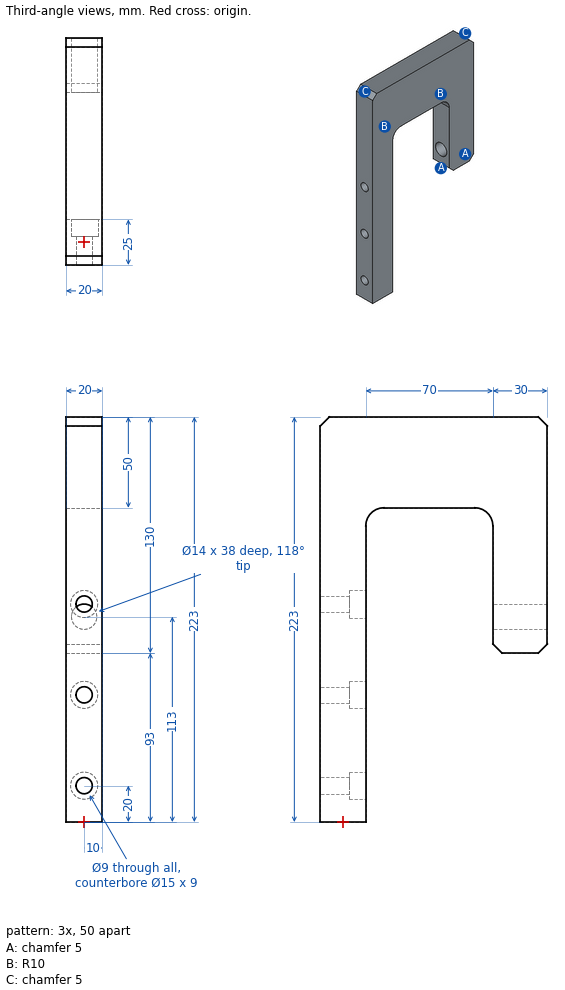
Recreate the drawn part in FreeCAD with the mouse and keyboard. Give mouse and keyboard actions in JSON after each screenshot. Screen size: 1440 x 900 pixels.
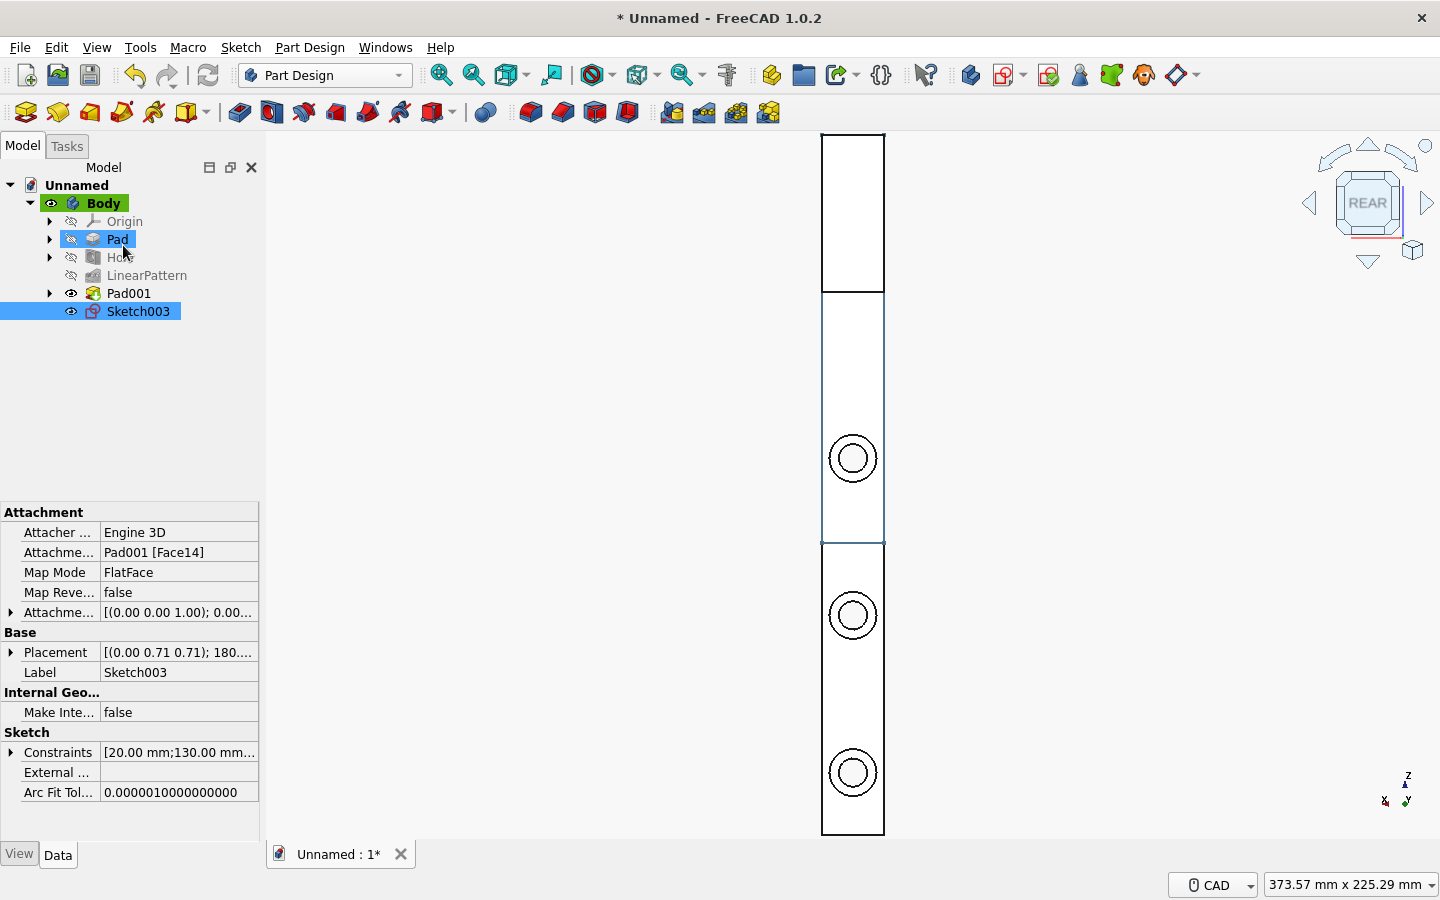
{"action": "left_click", "coordinate": [26, 112]}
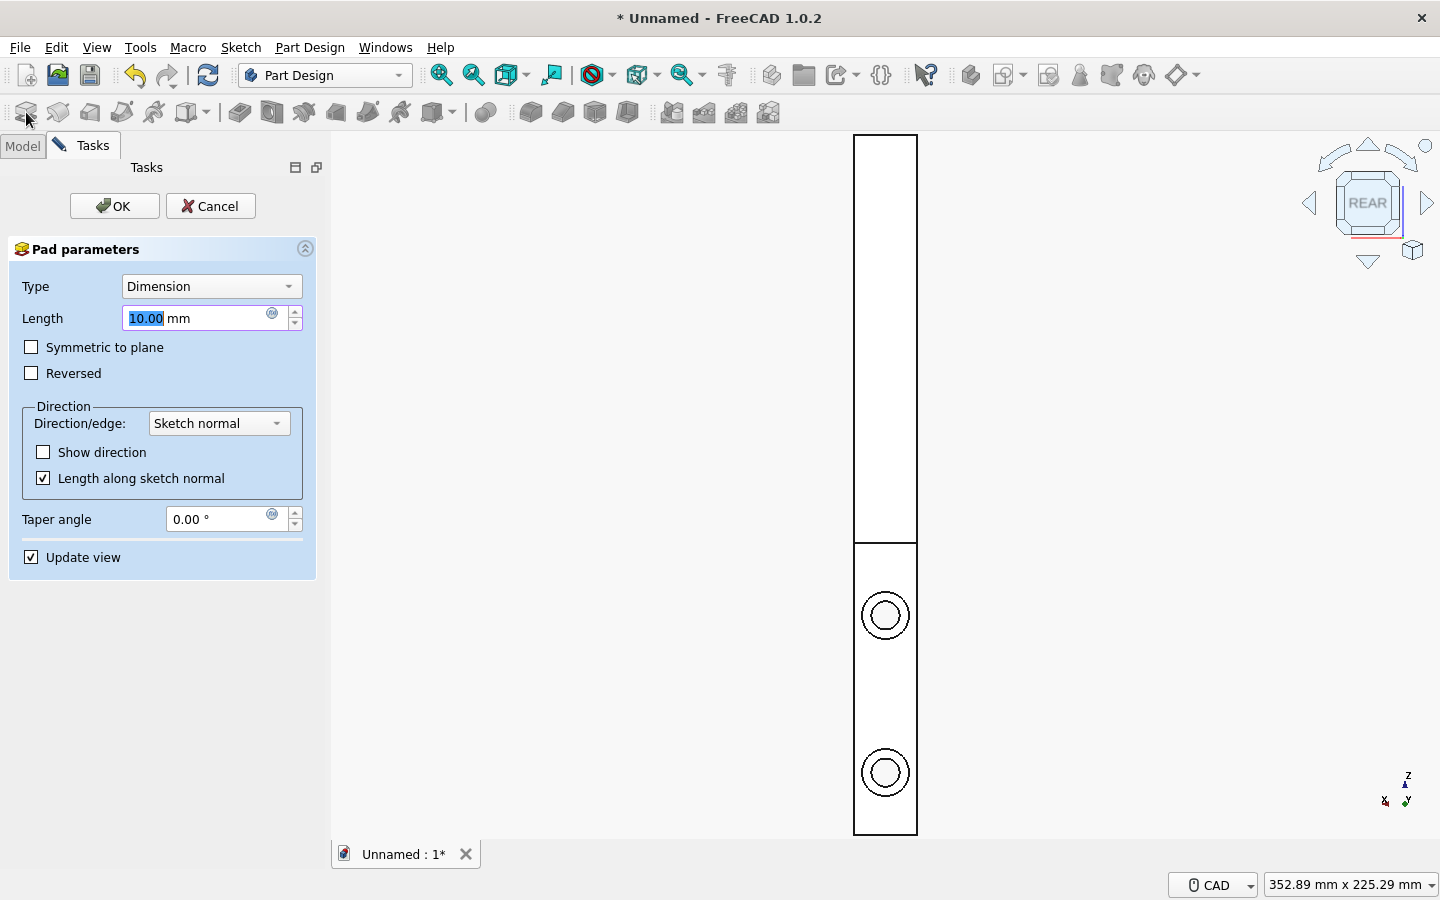
{"action": "type", "text": "30"}
{"action": "key", "text": "Tab"}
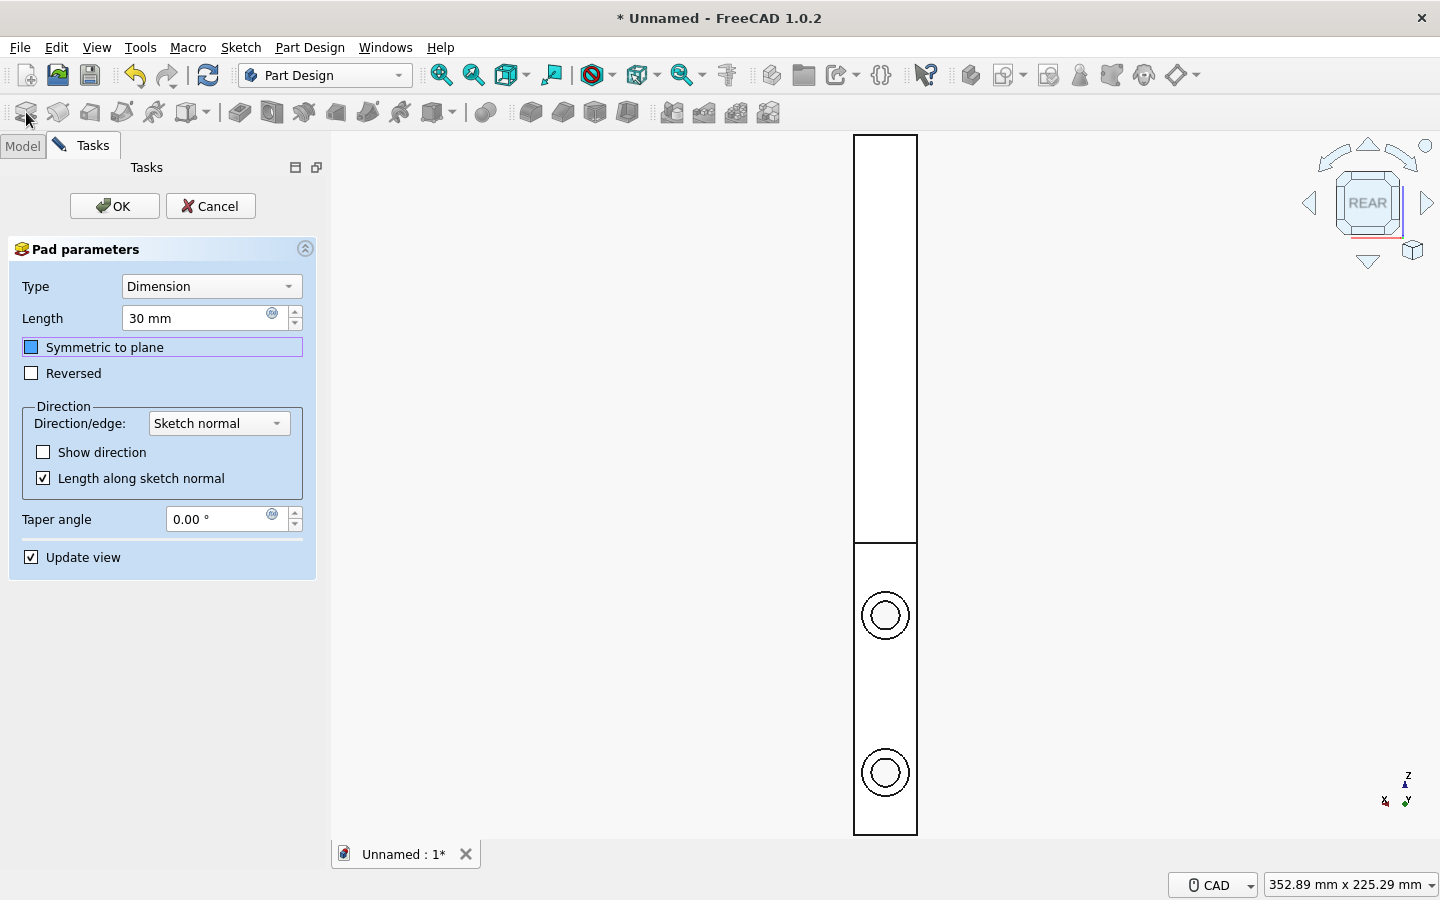
{"action": "left_click", "coordinate": [115, 206]}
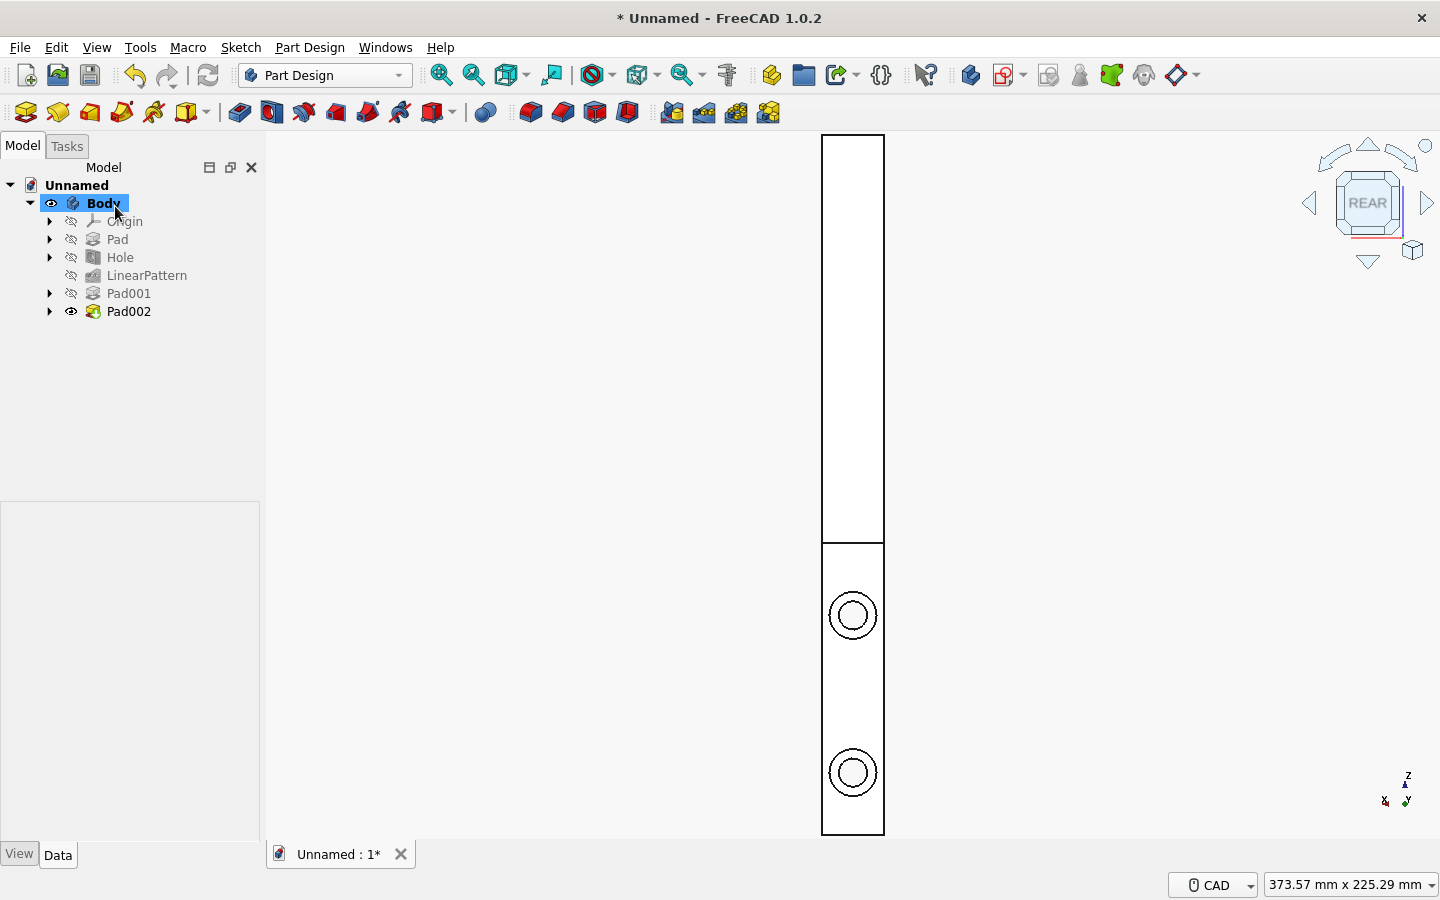
{"action": "left_click", "coordinate": [853, 221]}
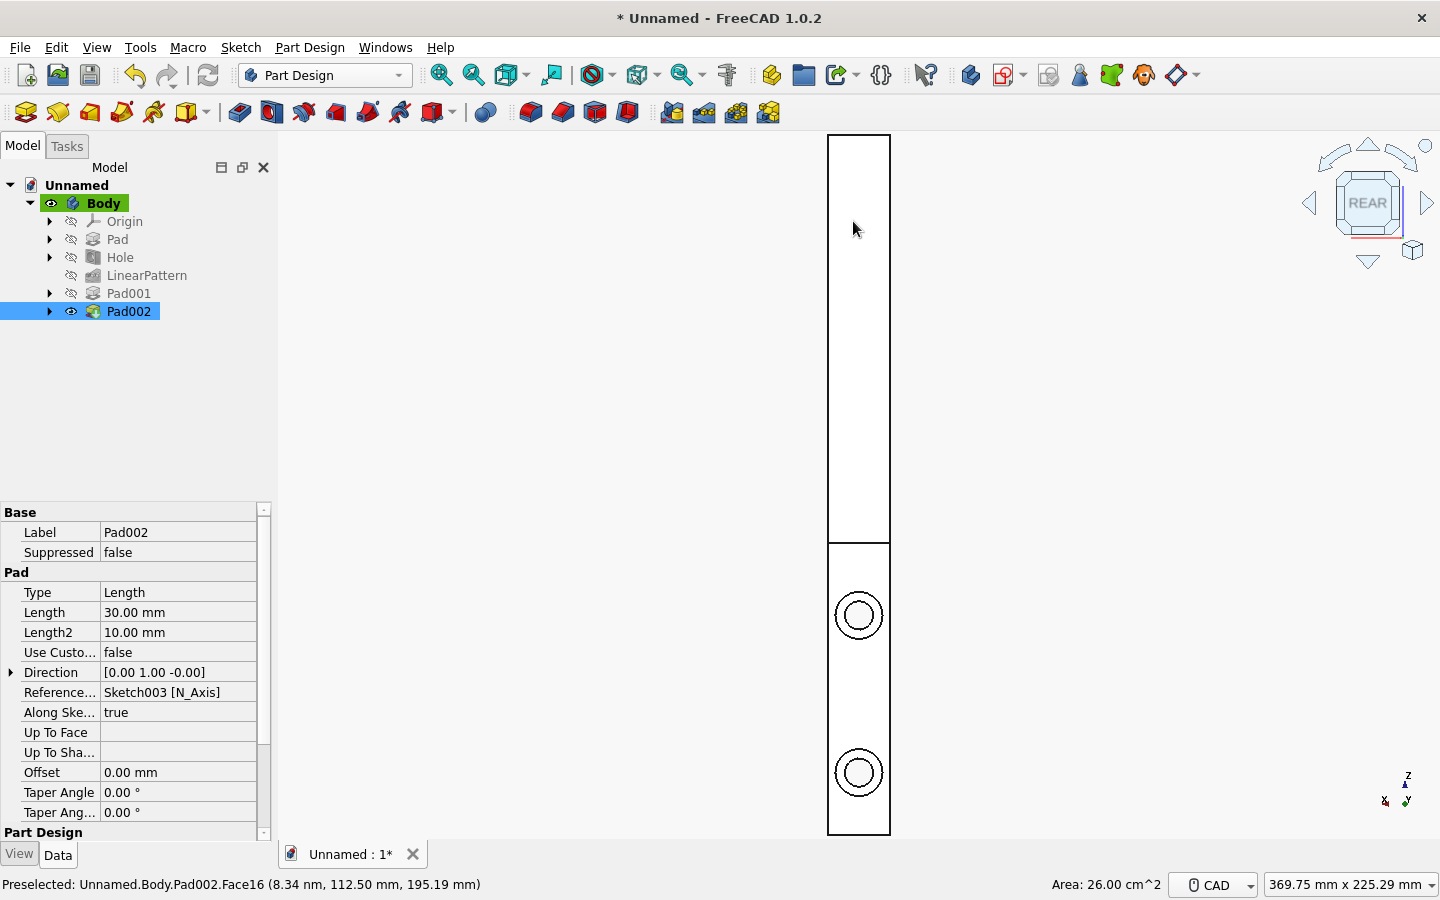
{"action": "left_click", "coordinate": [1004, 76]}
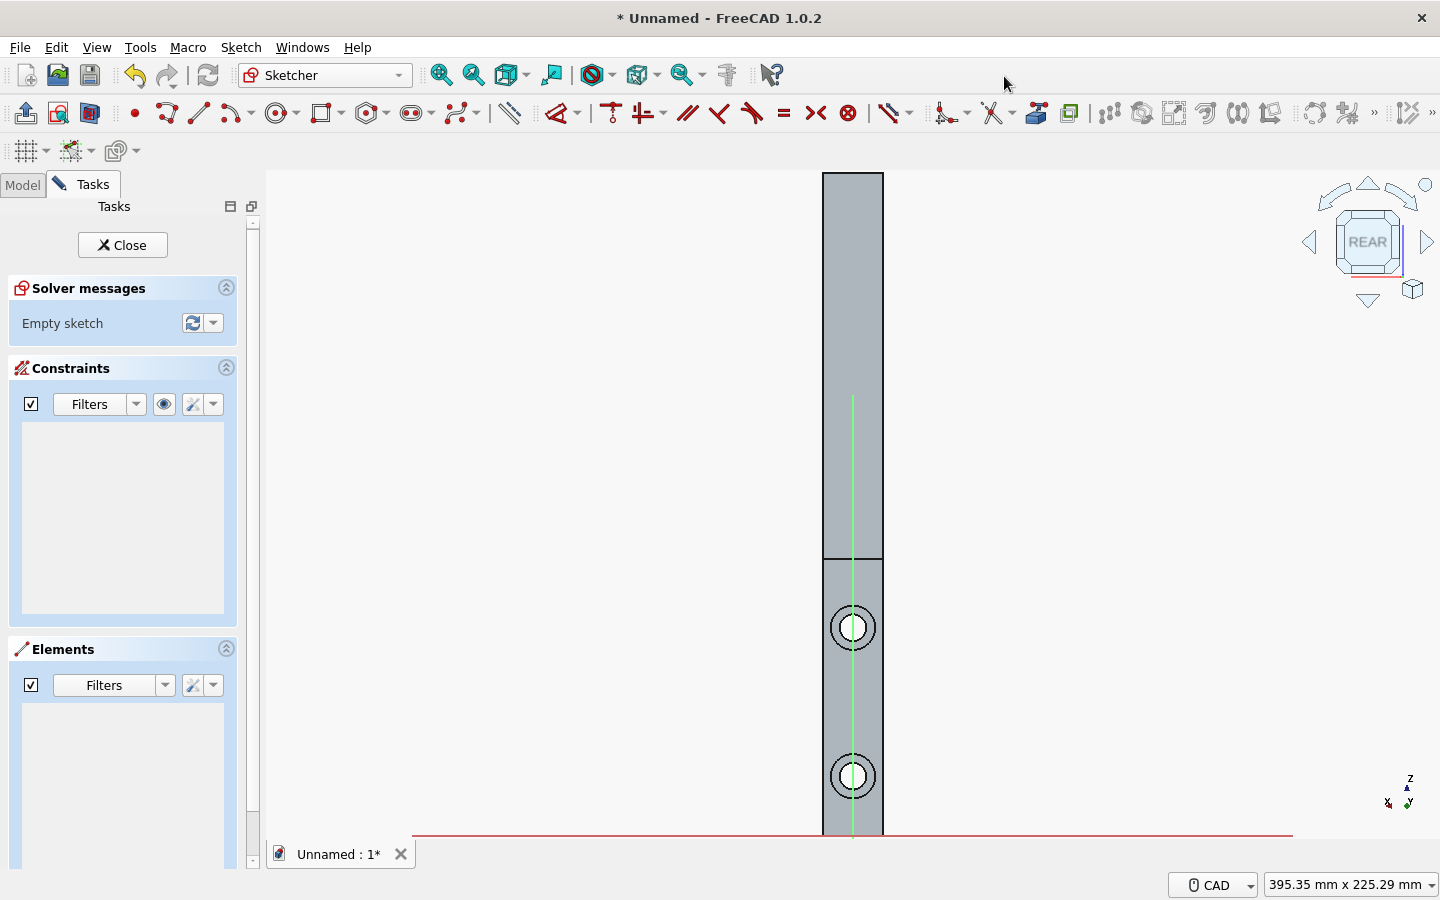
{"action": "scroll", "coordinate": [860, 500], "scroll_direction": "up", "scroll_amount": 12}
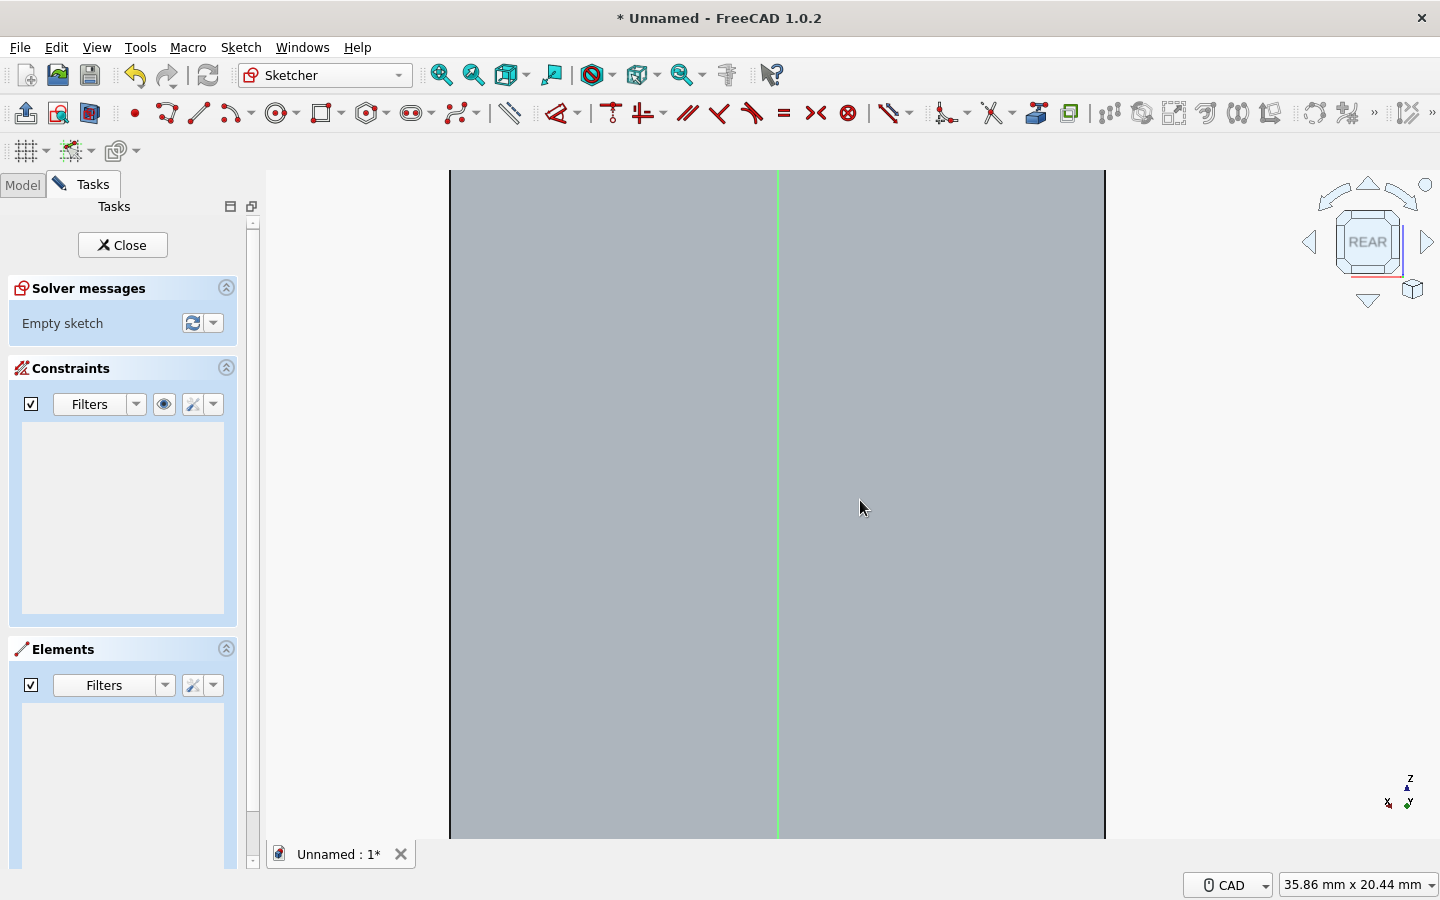
{"action": "left_click", "coordinate": [276, 114]}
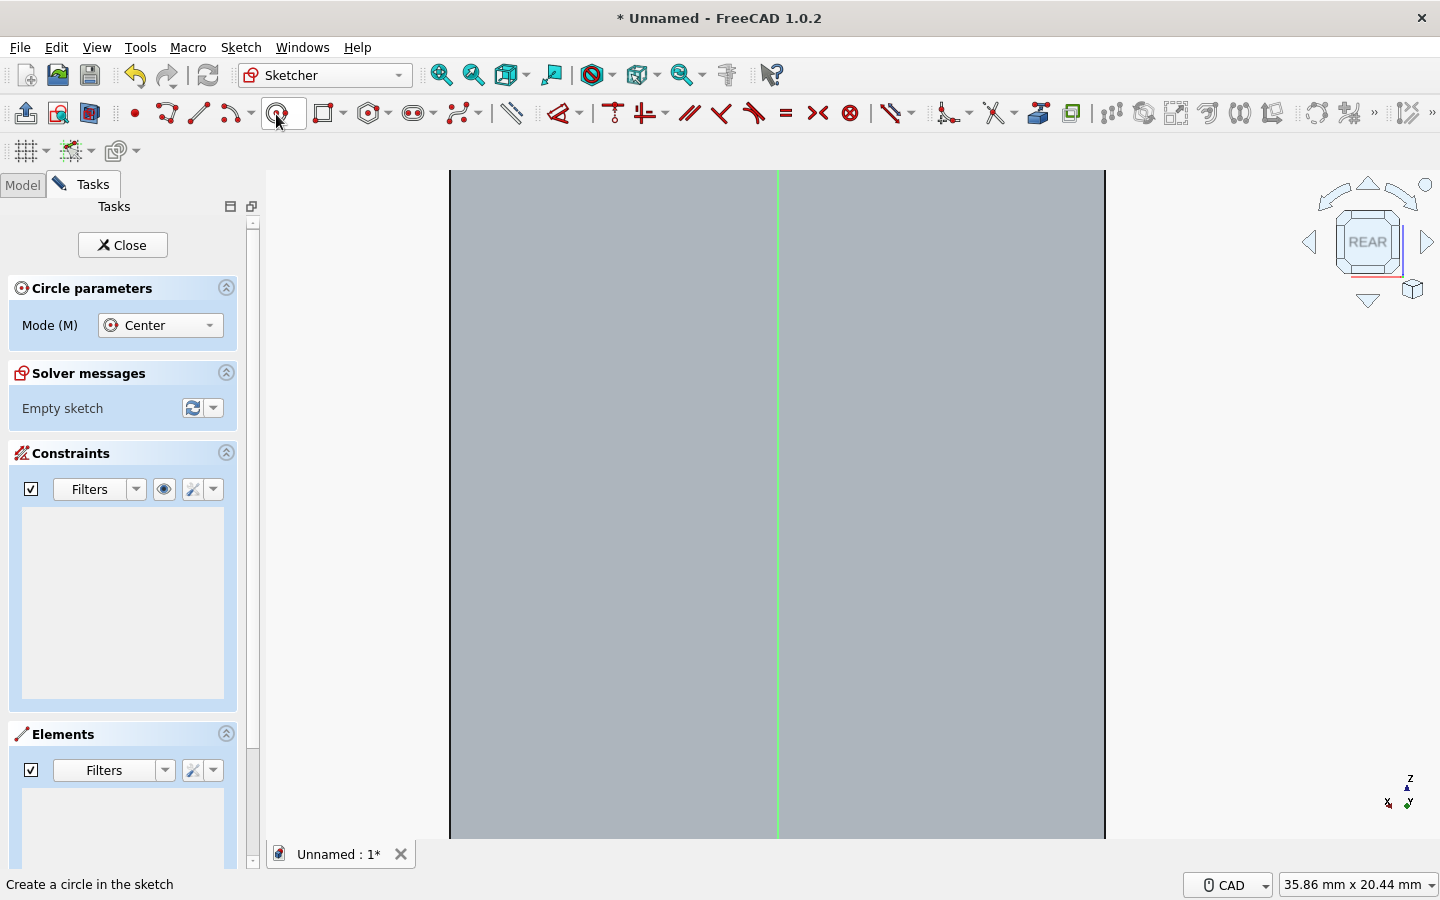
{"action": "left_click", "coordinate": [778, 496]}
{"action": "left_click", "coordinate": [940, 334]}
{"action": "key", "text": "Escape"}